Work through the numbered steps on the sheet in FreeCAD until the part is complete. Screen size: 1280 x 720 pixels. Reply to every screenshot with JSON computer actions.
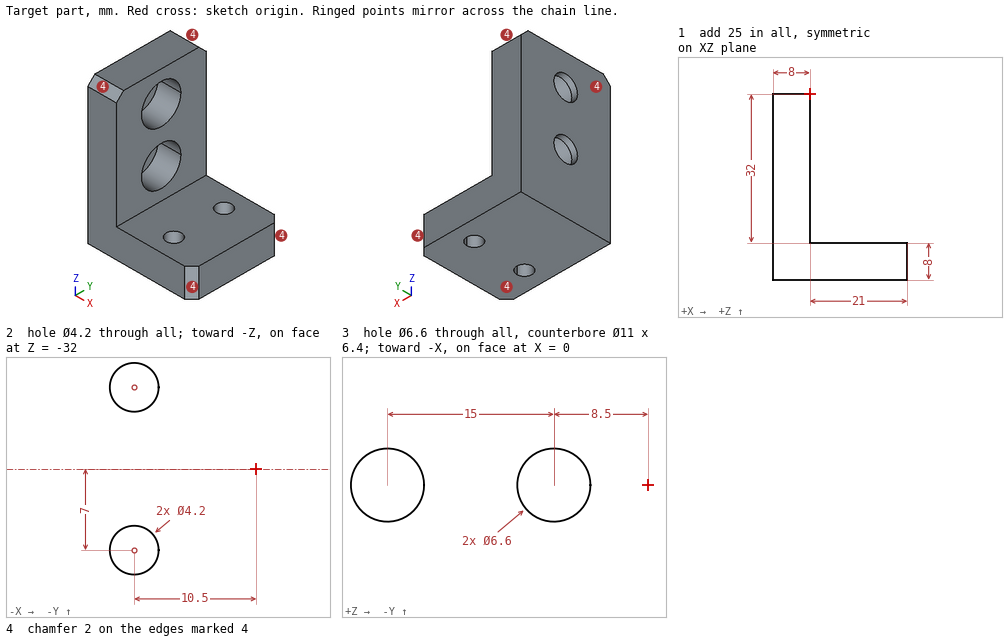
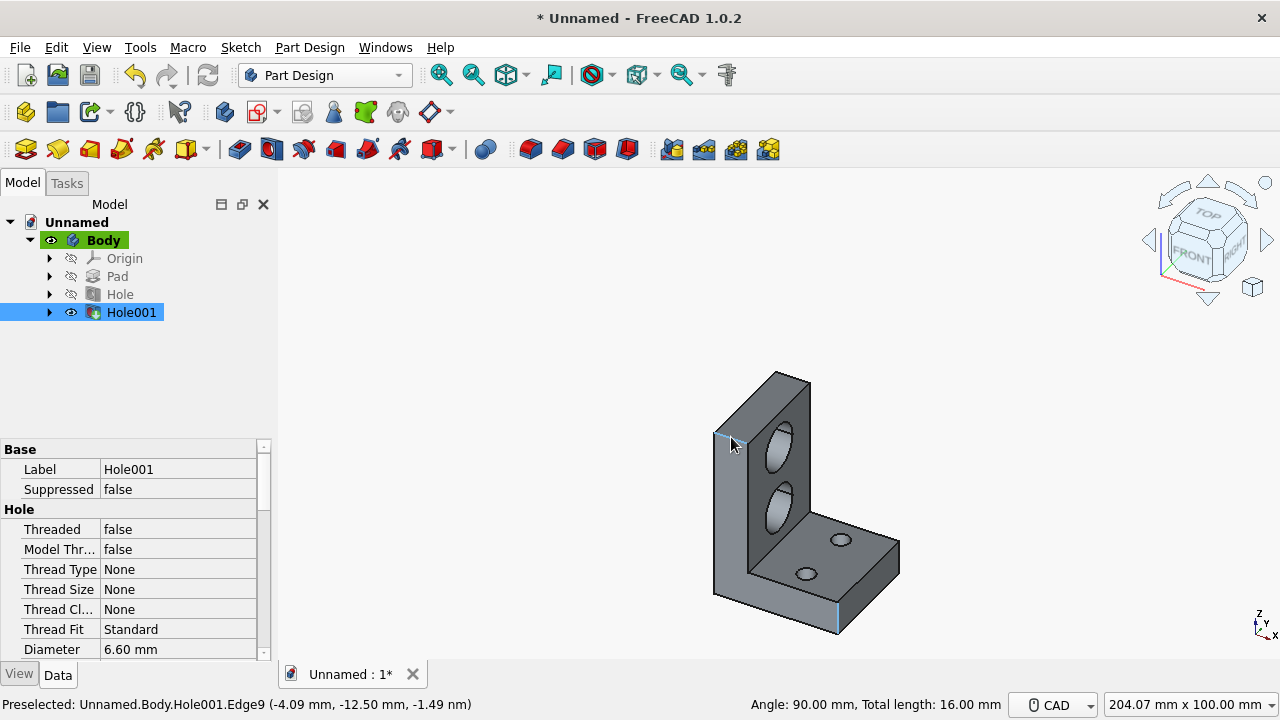
{"action": "key", "text": "0"}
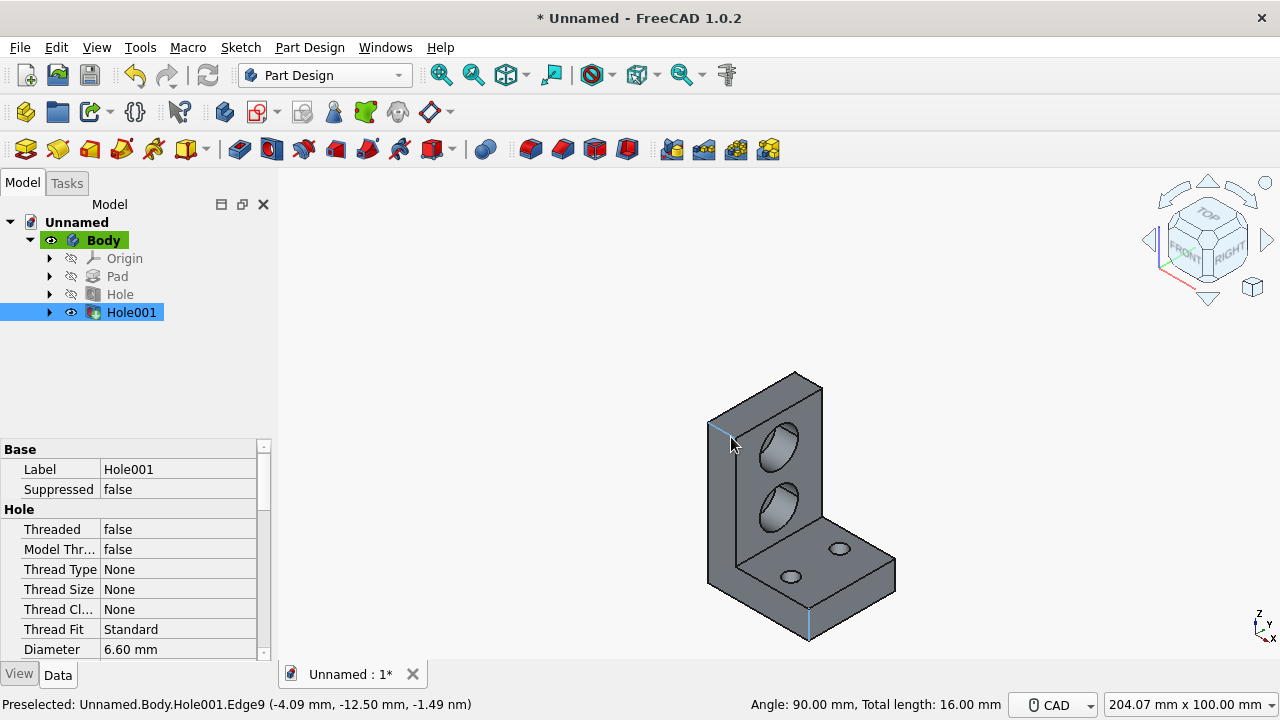
{"action": "key", "text": "2"}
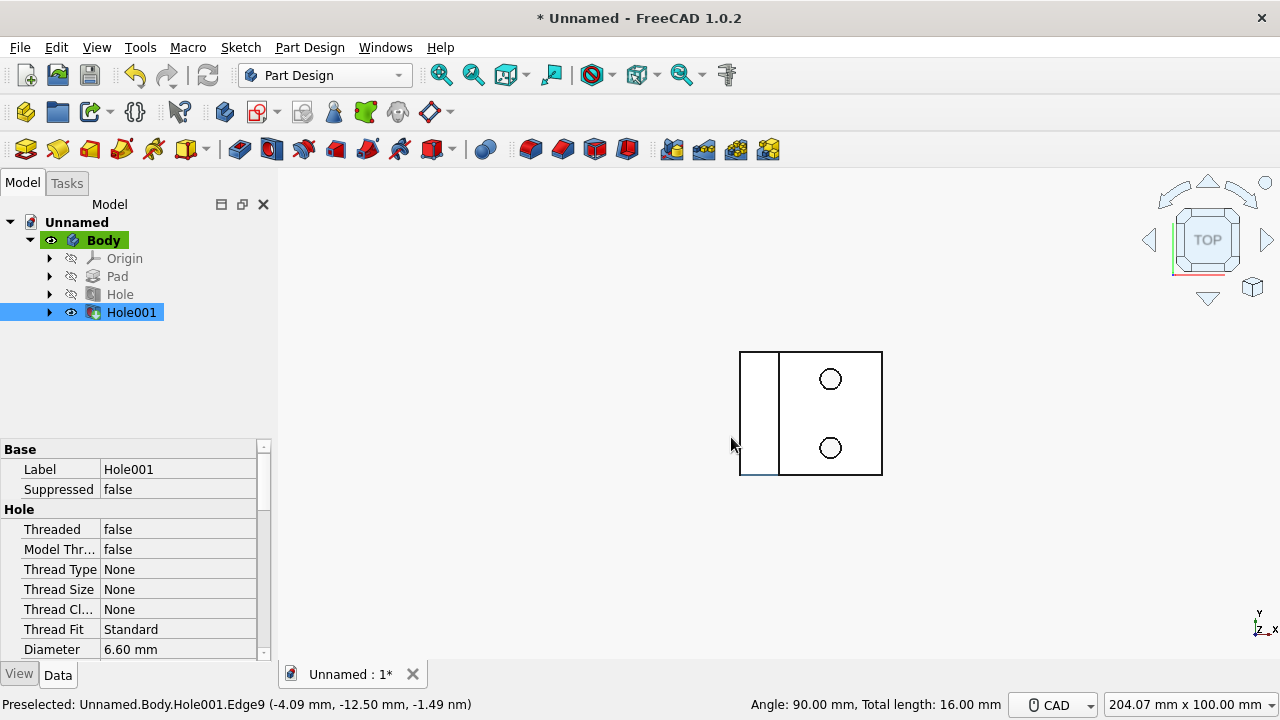
{"action": "key", "text": "v f"}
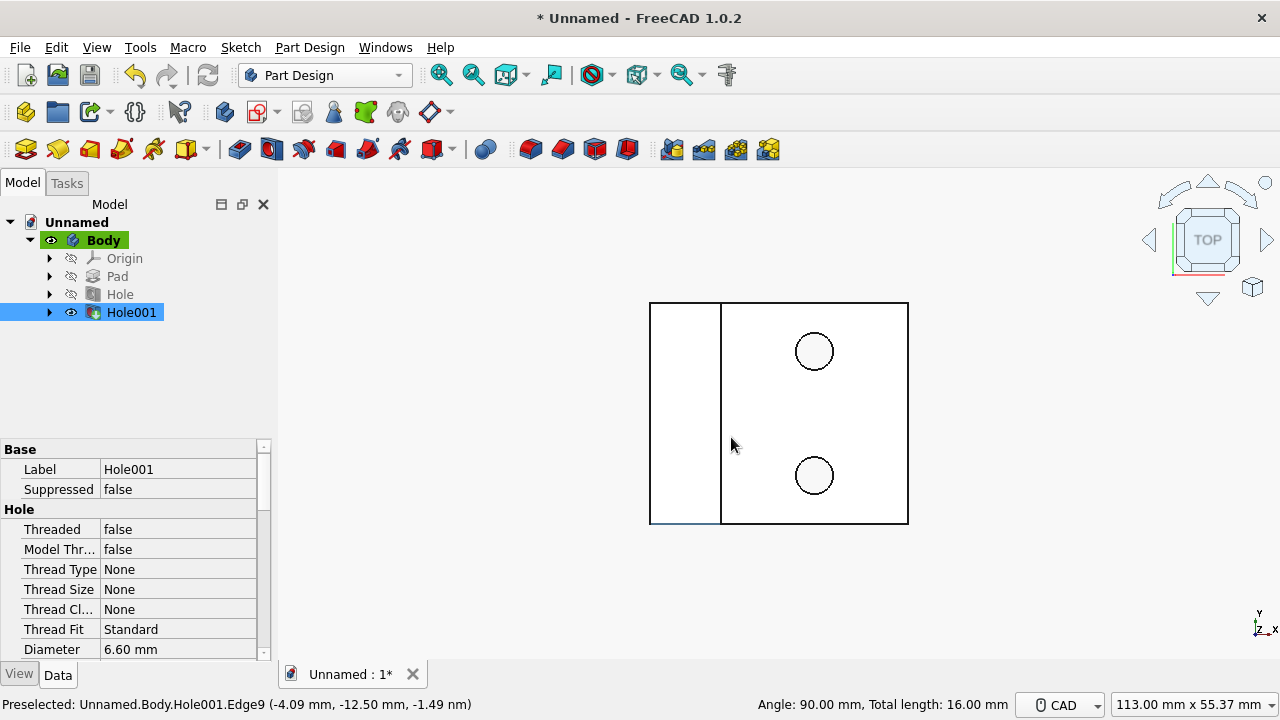
{"action": "left_click", "coordinate": [686, 302], "text": "ctrl"}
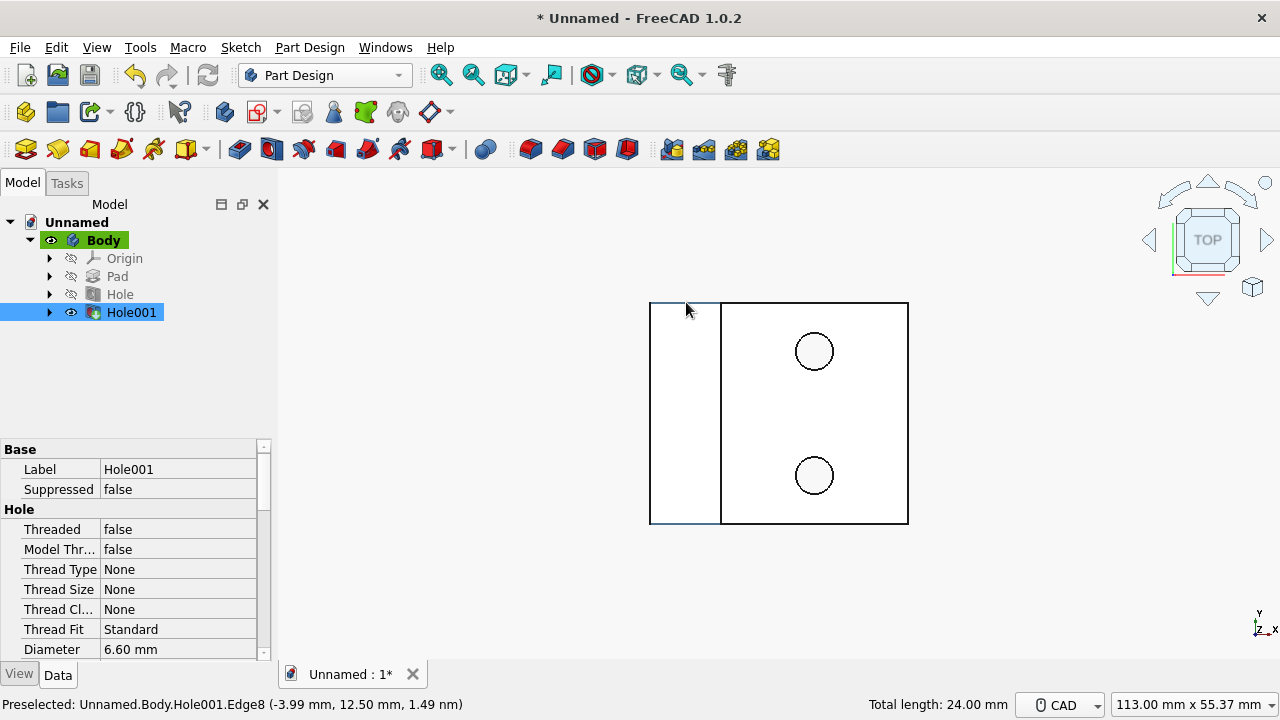
{"action": "key", "text": "1"}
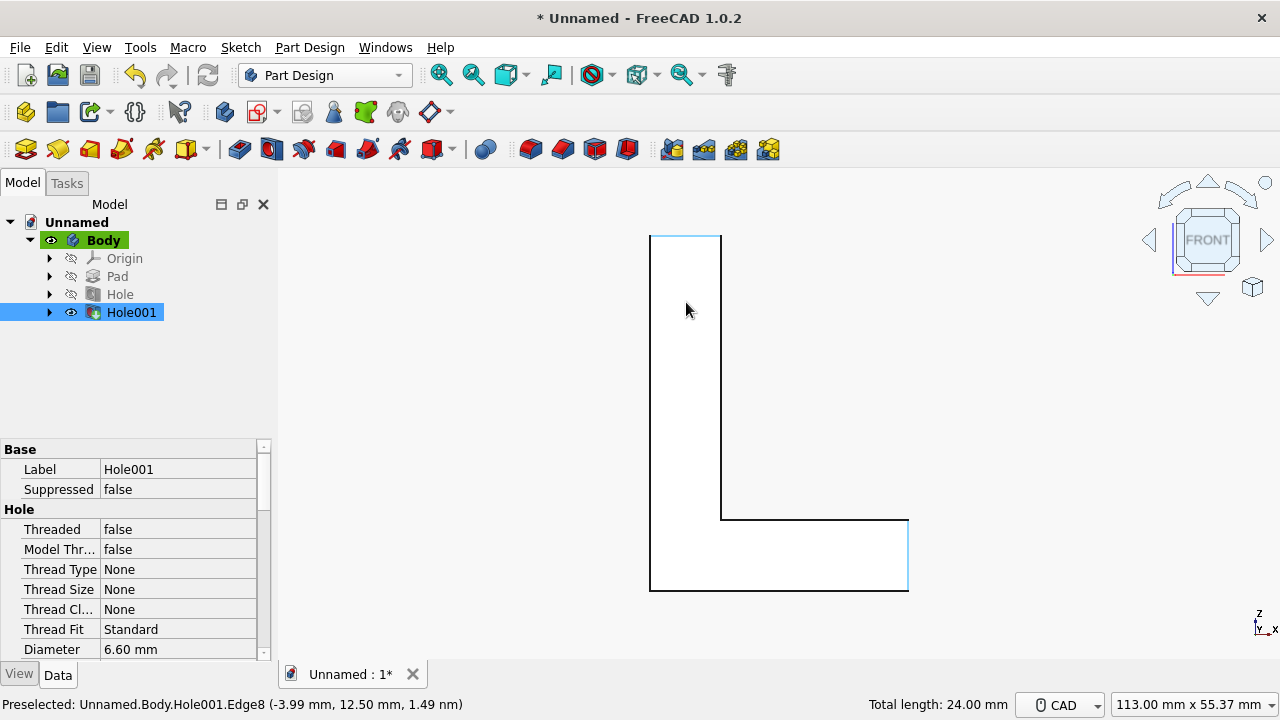
{"action": "key", "text": "3"}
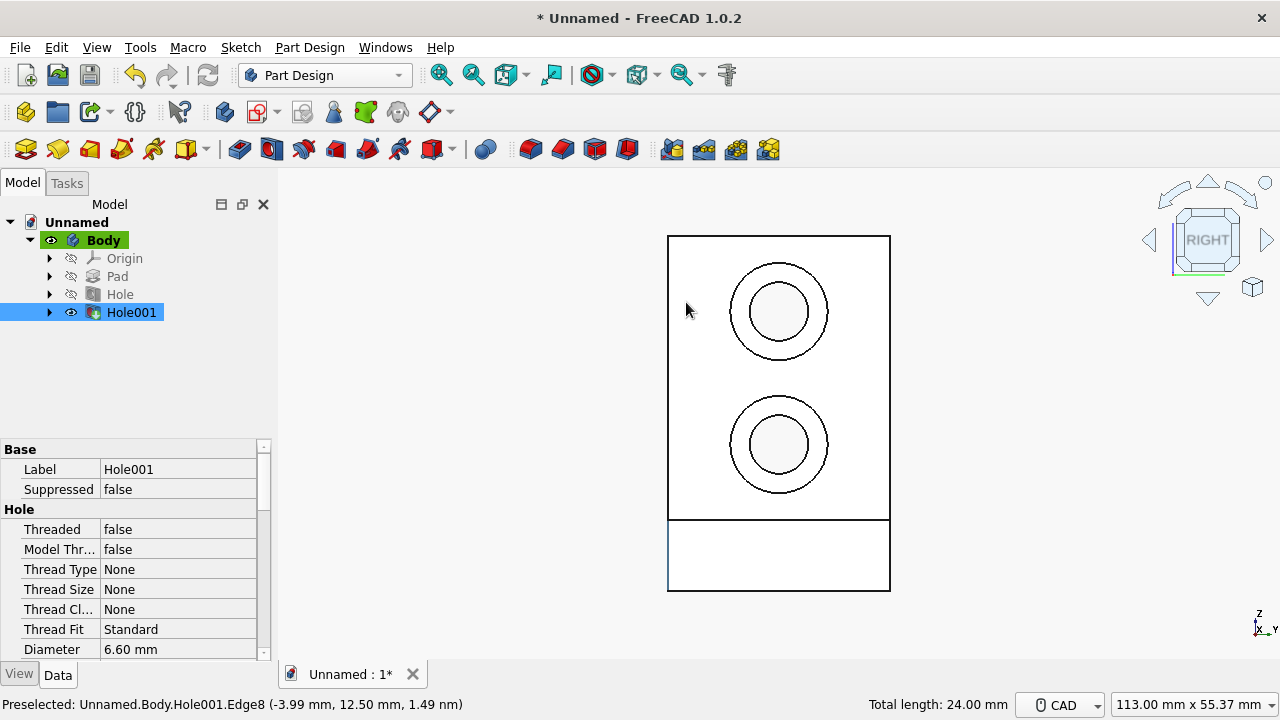
{"action": "left_click", "coordinate": [890, 554], "text": "ctrl"}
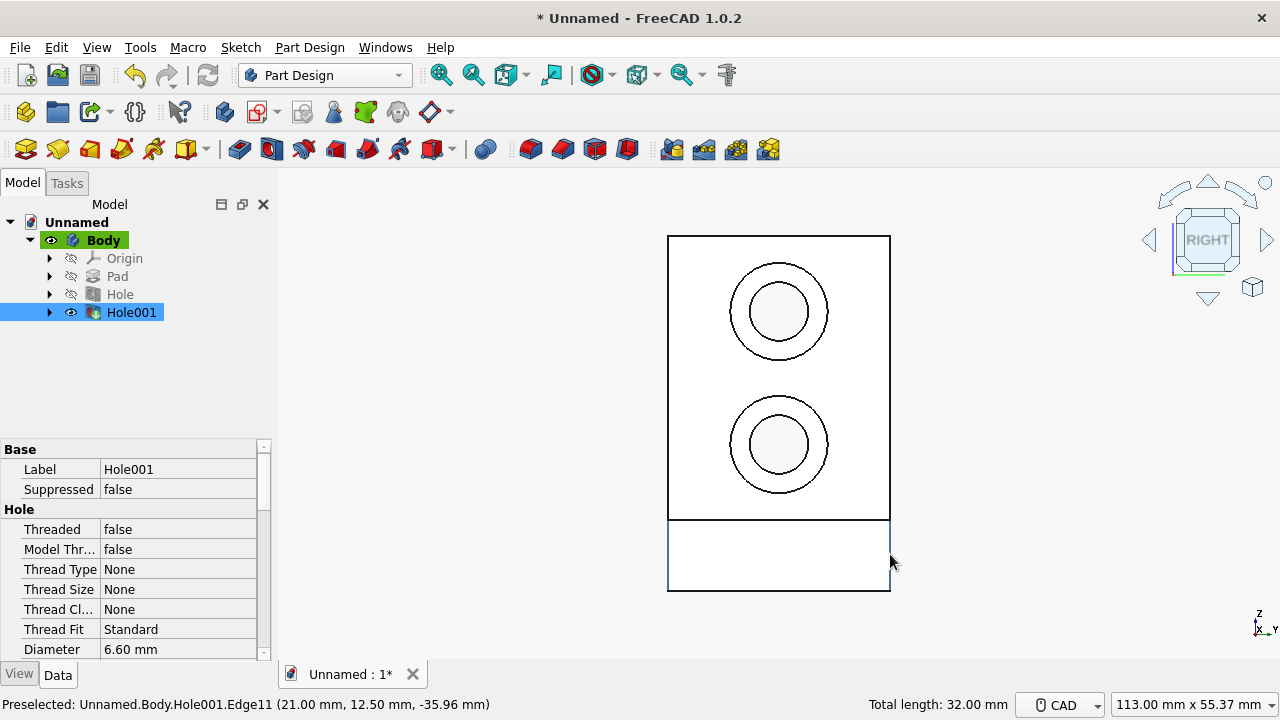
{"action": "left_click", "coordinate": [564, 150]}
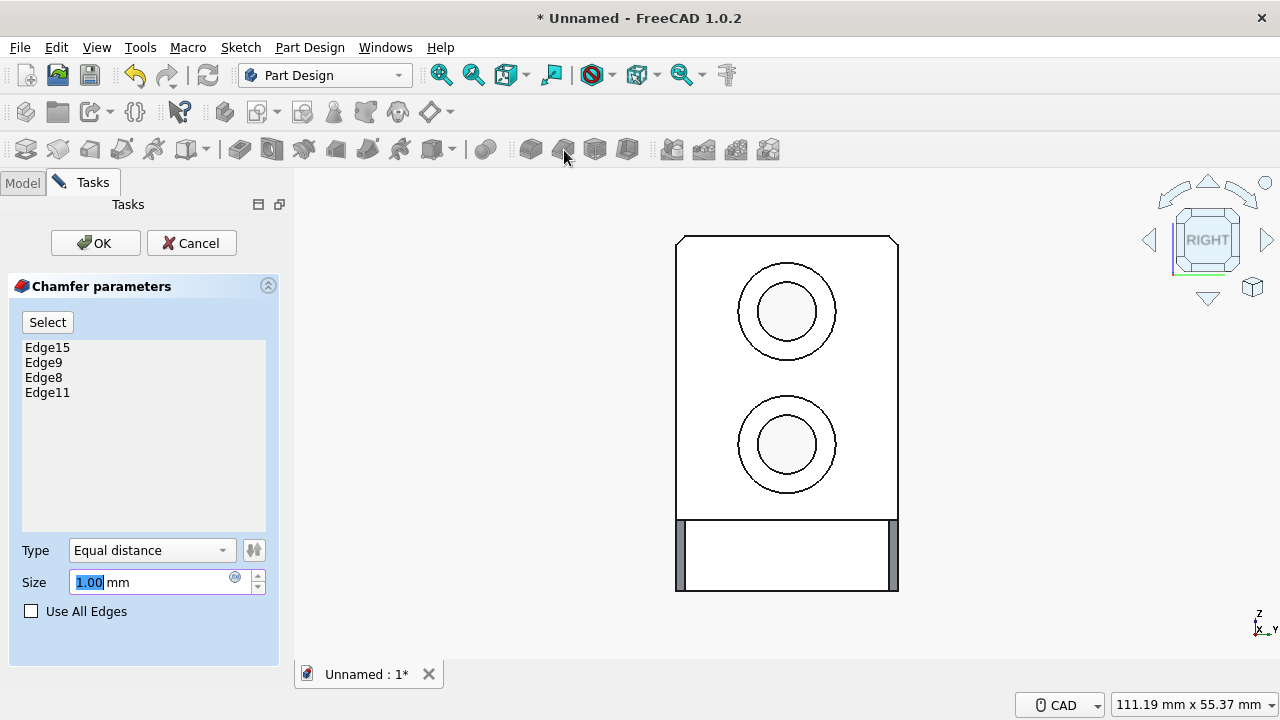
{"action": "type", "text": "2"}
{"action": "key", "text": "Tab"}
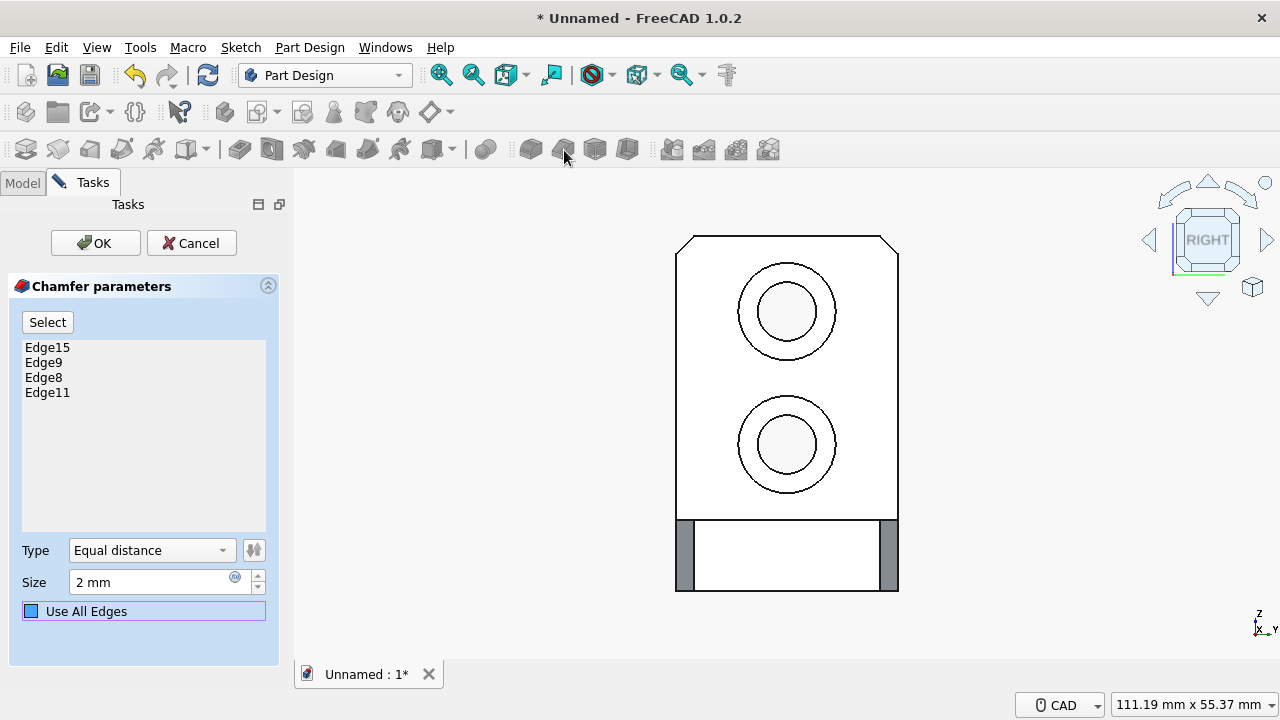
{"action": "left_click", "coordinate": [96, 243]}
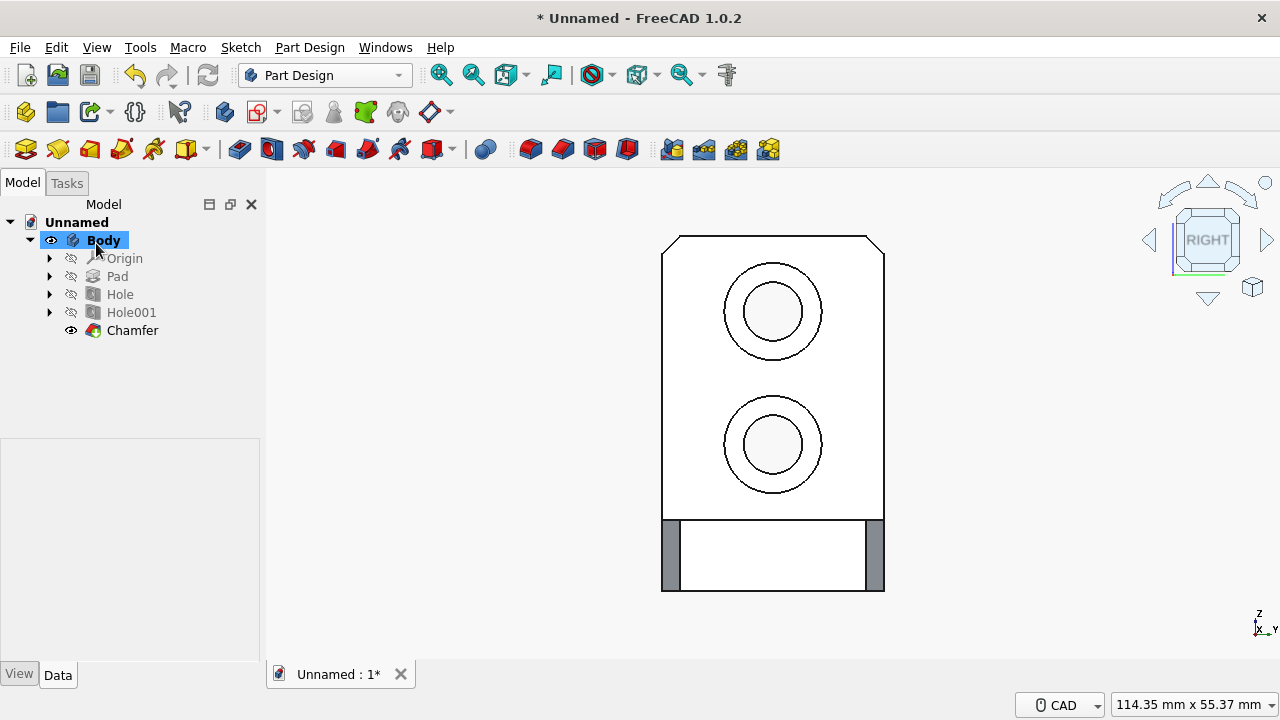
{"action": "key", "text": "0"}